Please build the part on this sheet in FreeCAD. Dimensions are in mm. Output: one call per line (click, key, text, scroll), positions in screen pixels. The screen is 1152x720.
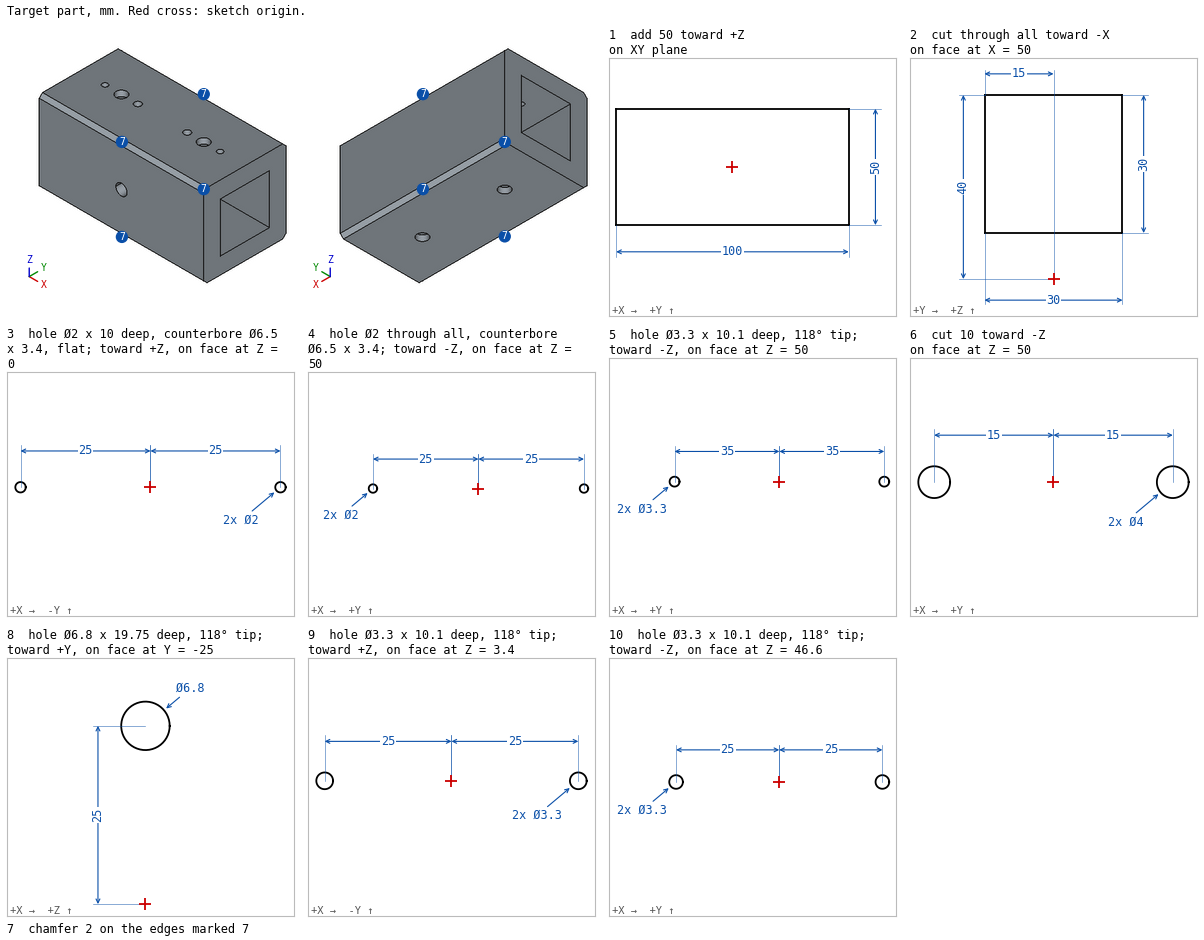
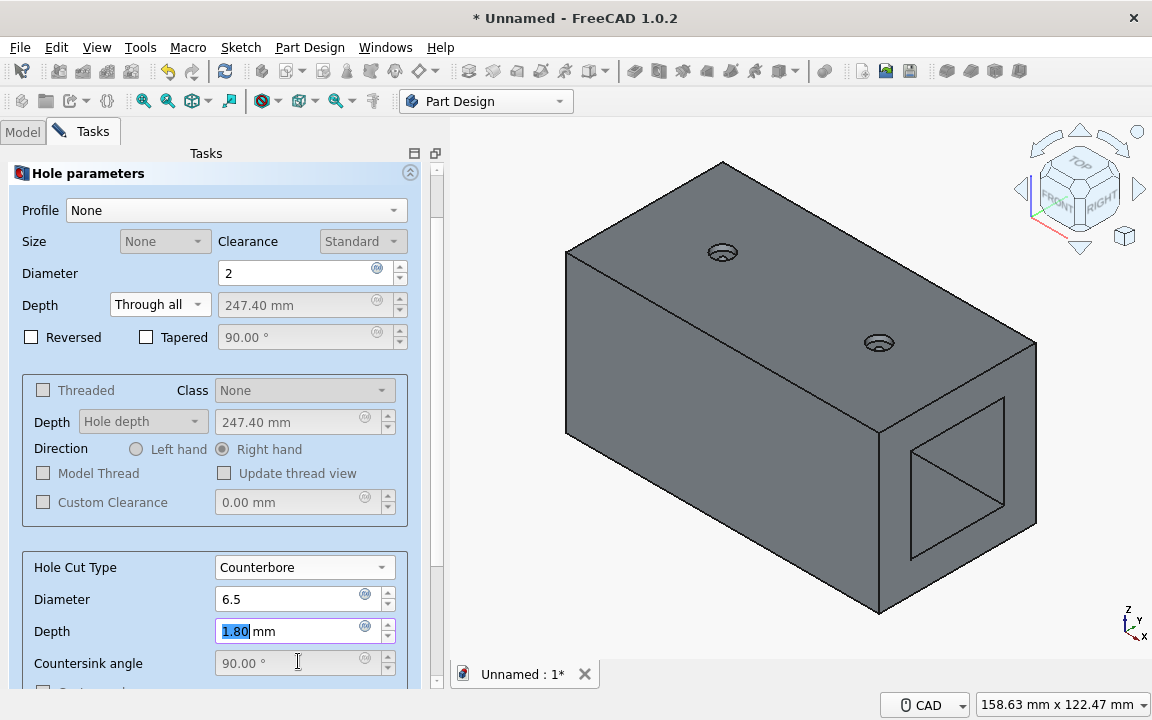
text(3.4)
key(Tab)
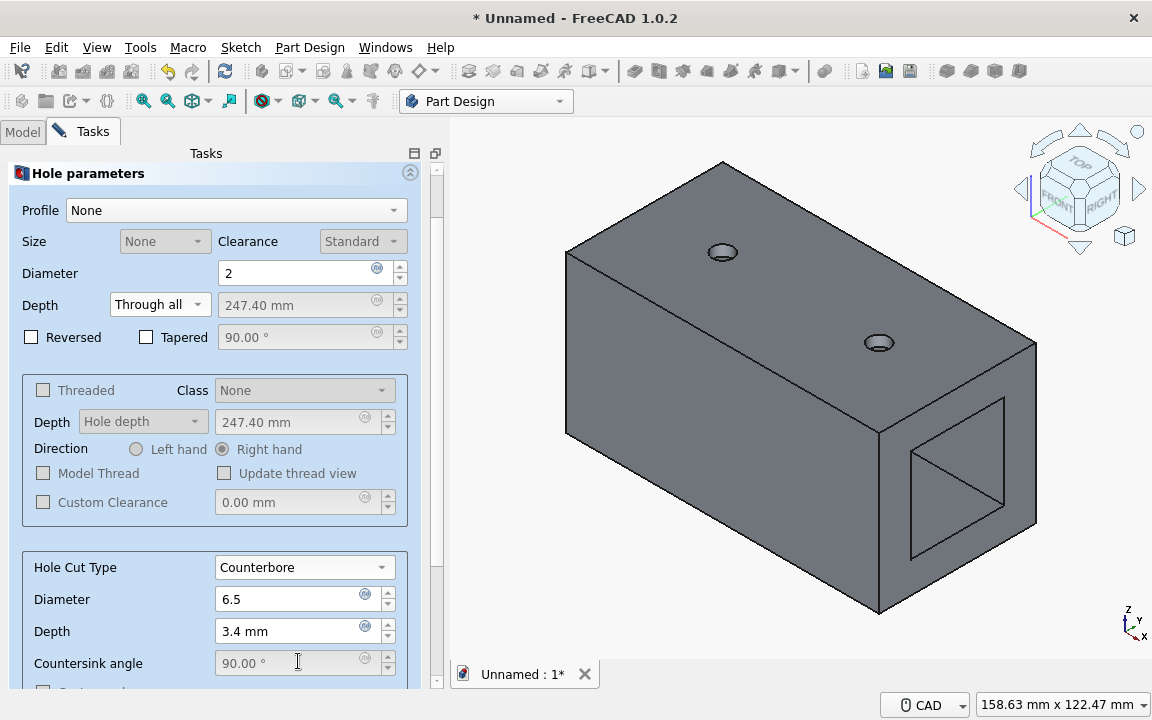
scroll(437, 426, up, 2)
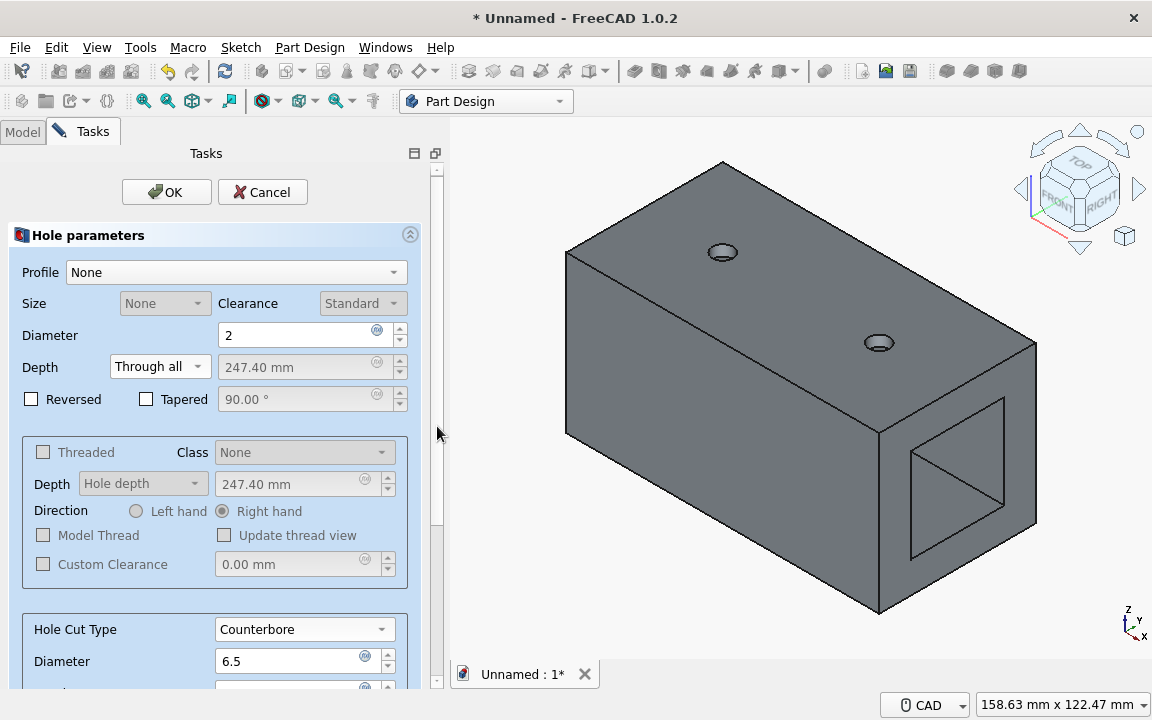
click(167, 192)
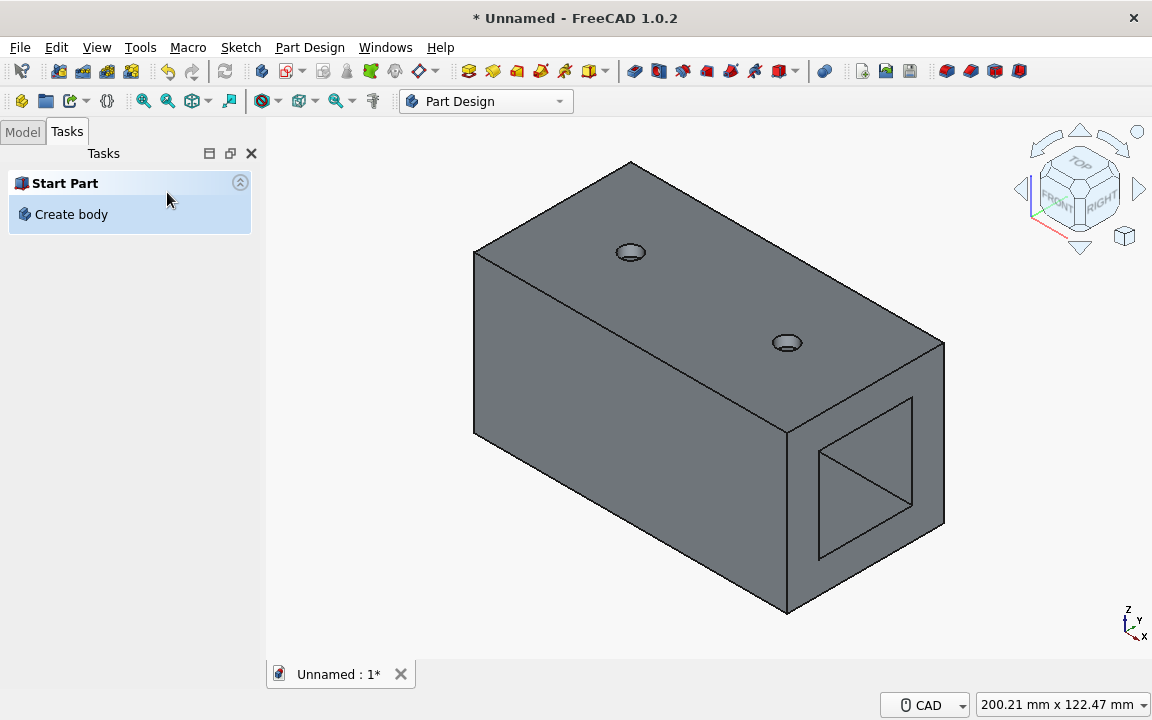
click(709, 297)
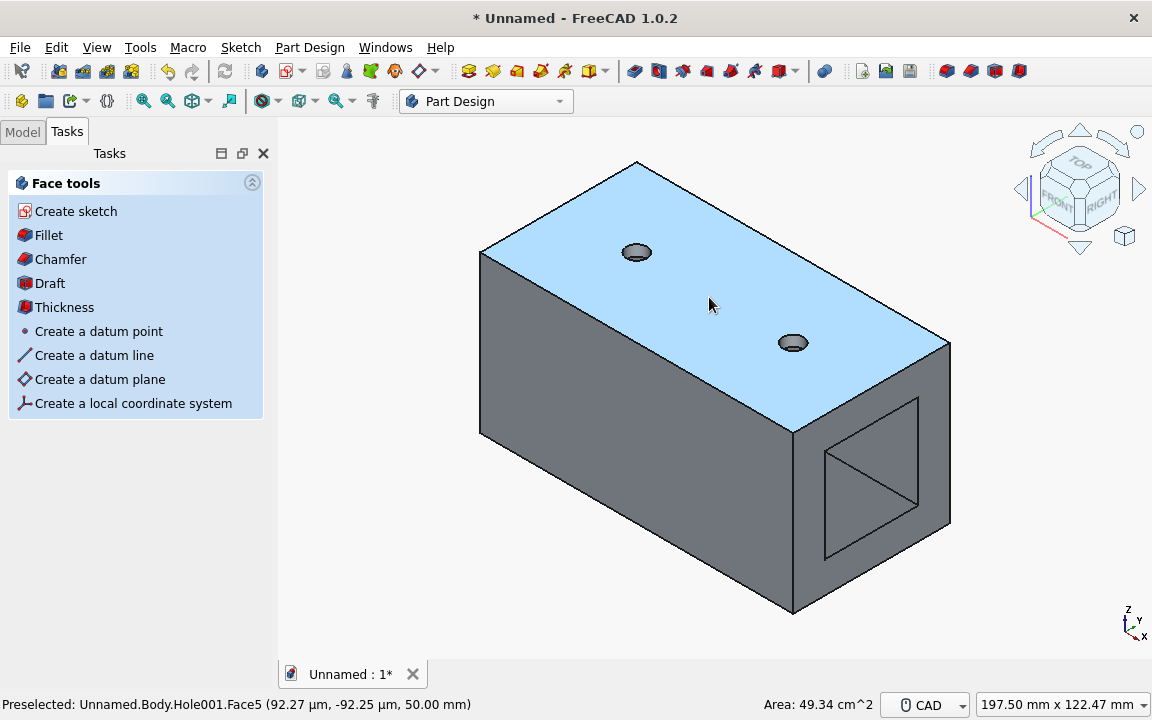
click(286, 72)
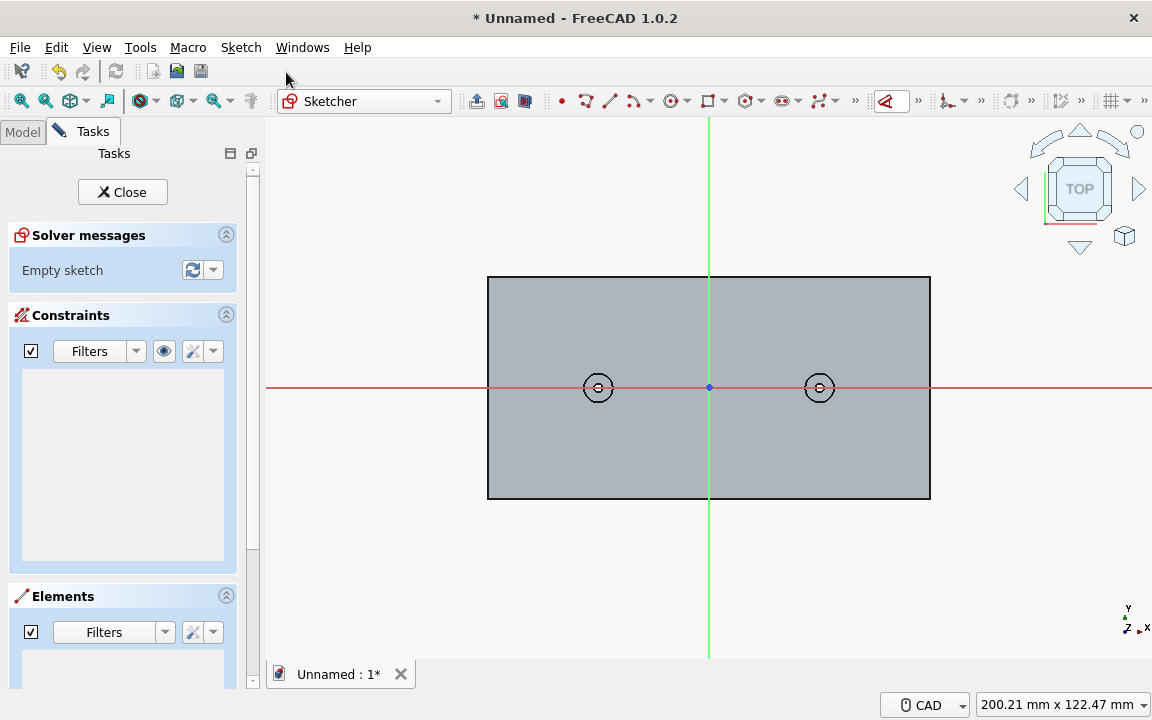
scroll(848, 388, up, 2)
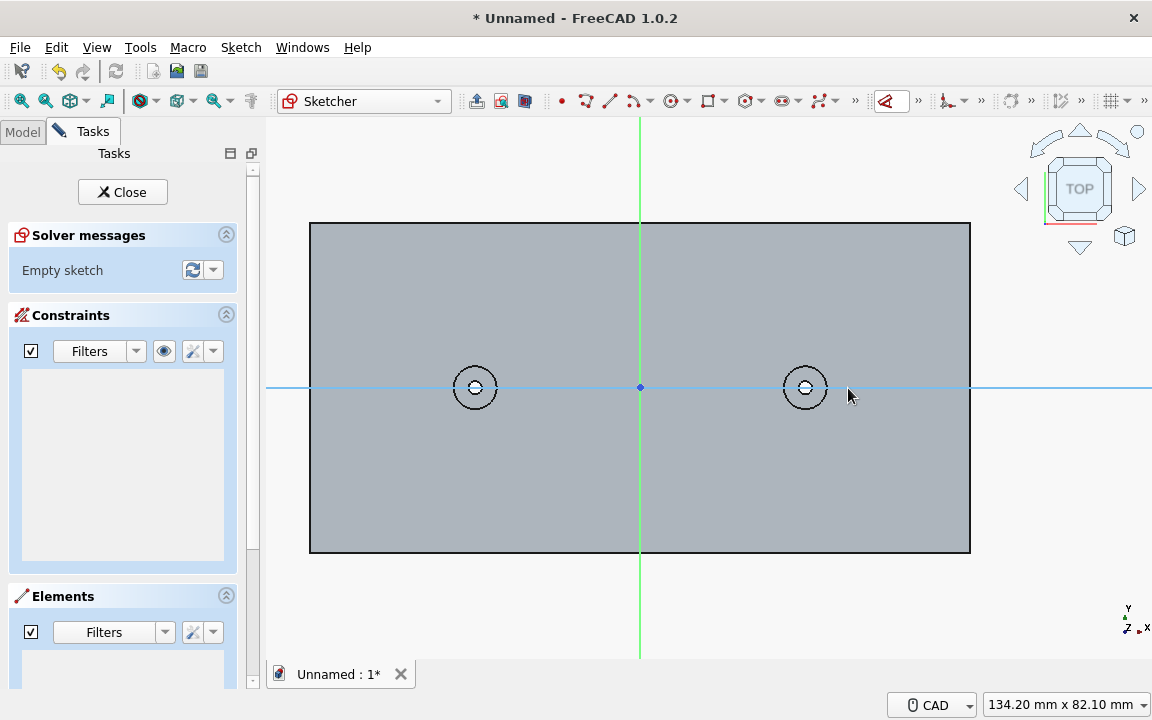
key(g)
key(c)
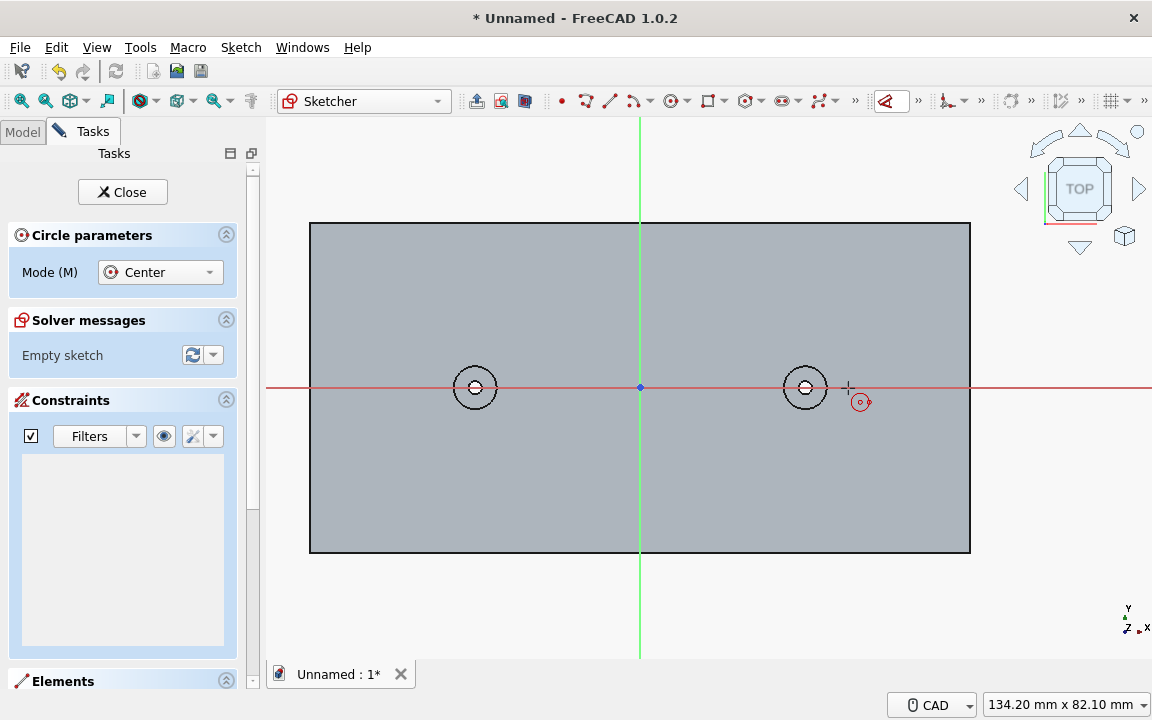
scroll(409, 388, up, 4)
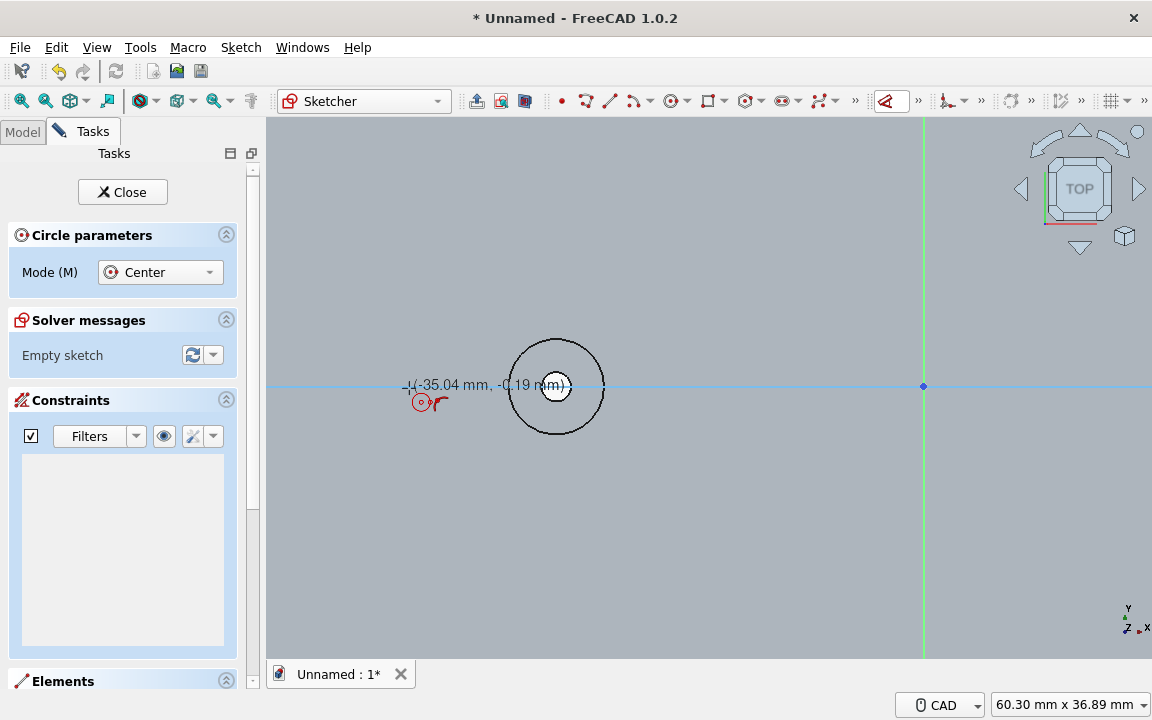
click(409, 387)
move(426, 370)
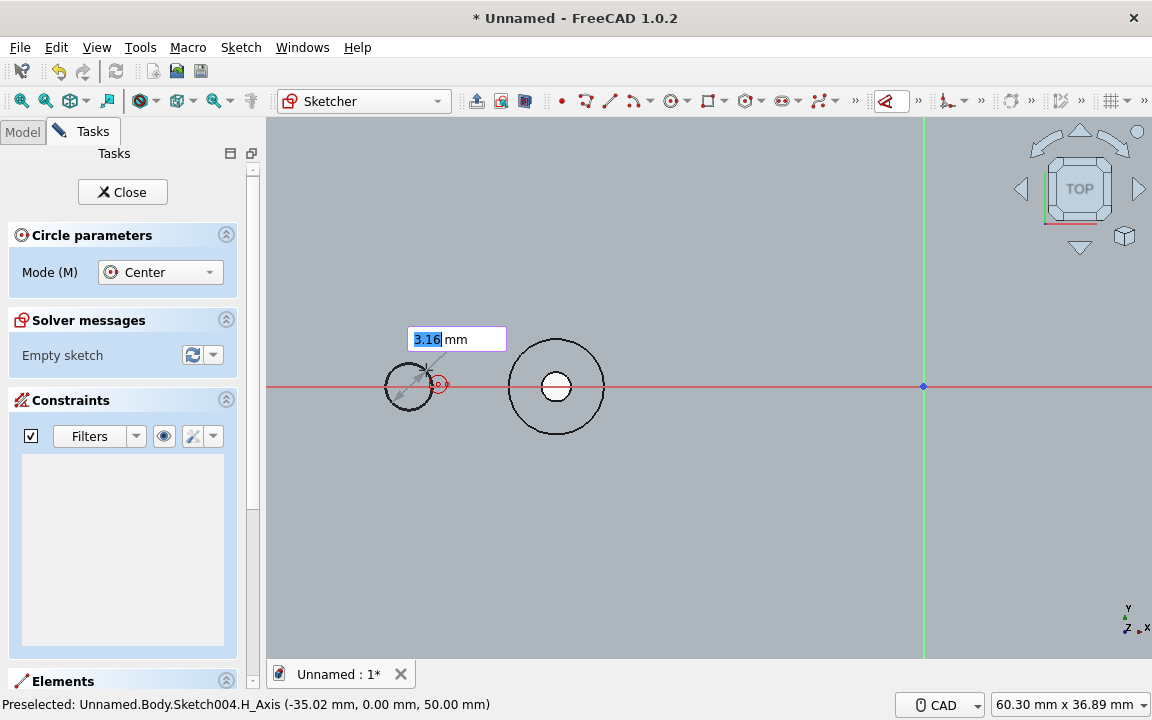
text(3.3)
key(Return)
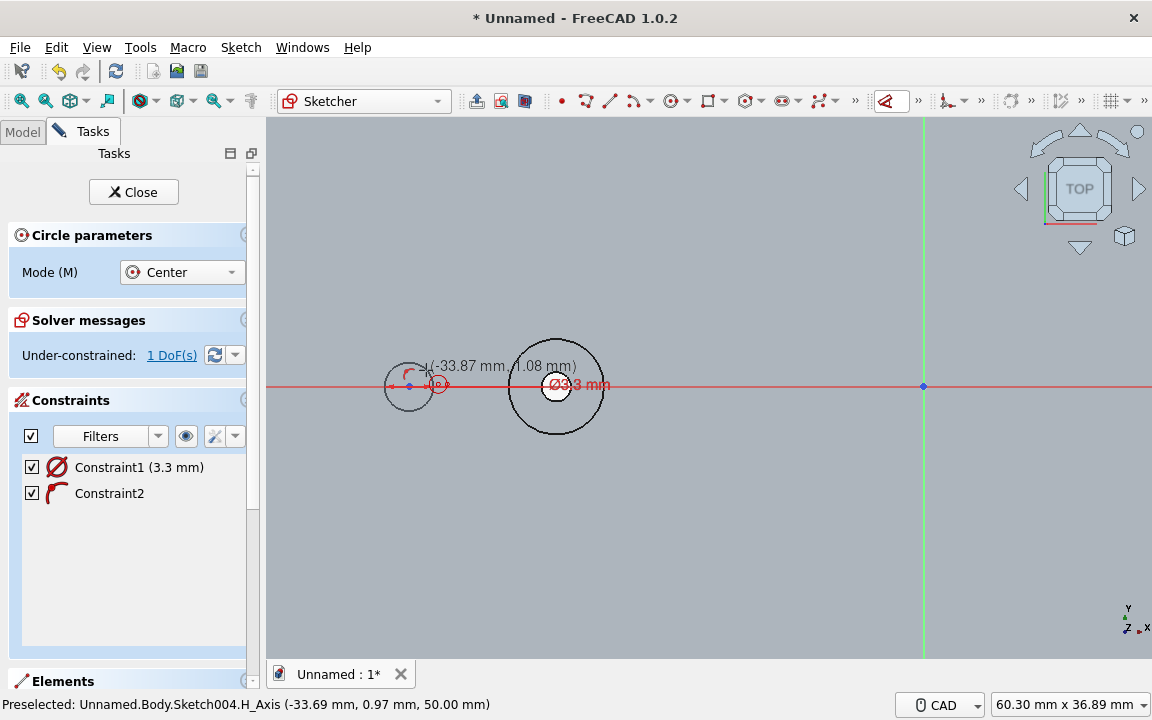
scroll(410, 389, down, 4)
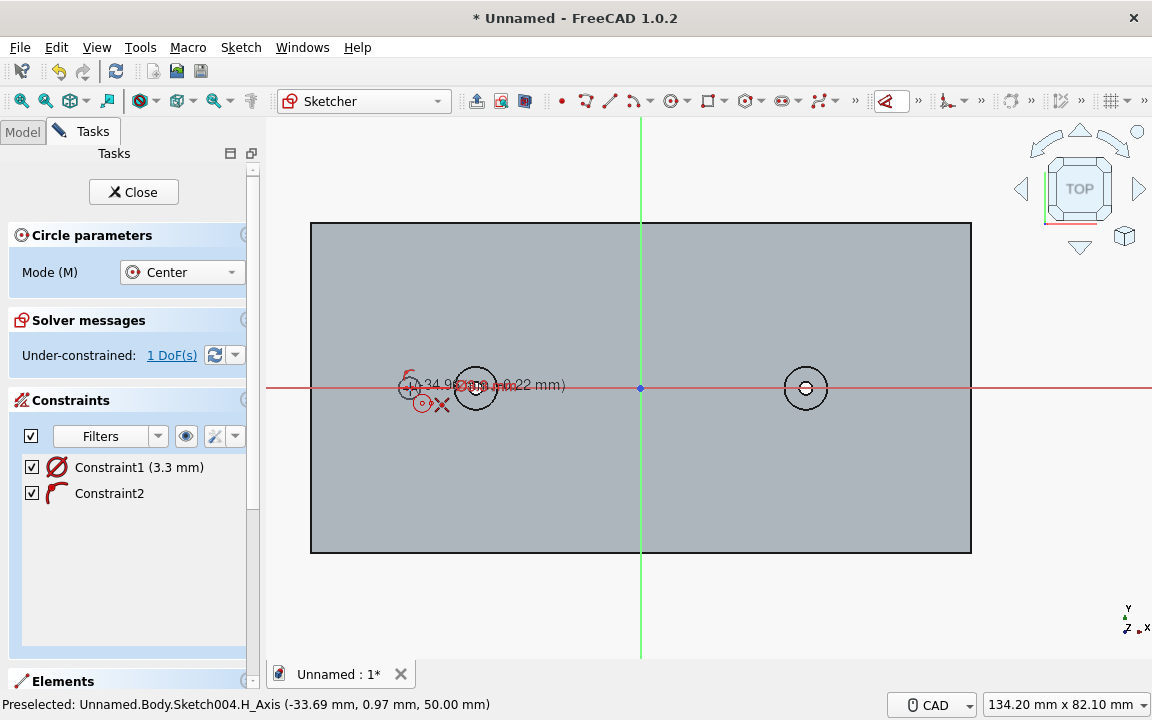
scroll(872, 388, up, 4)